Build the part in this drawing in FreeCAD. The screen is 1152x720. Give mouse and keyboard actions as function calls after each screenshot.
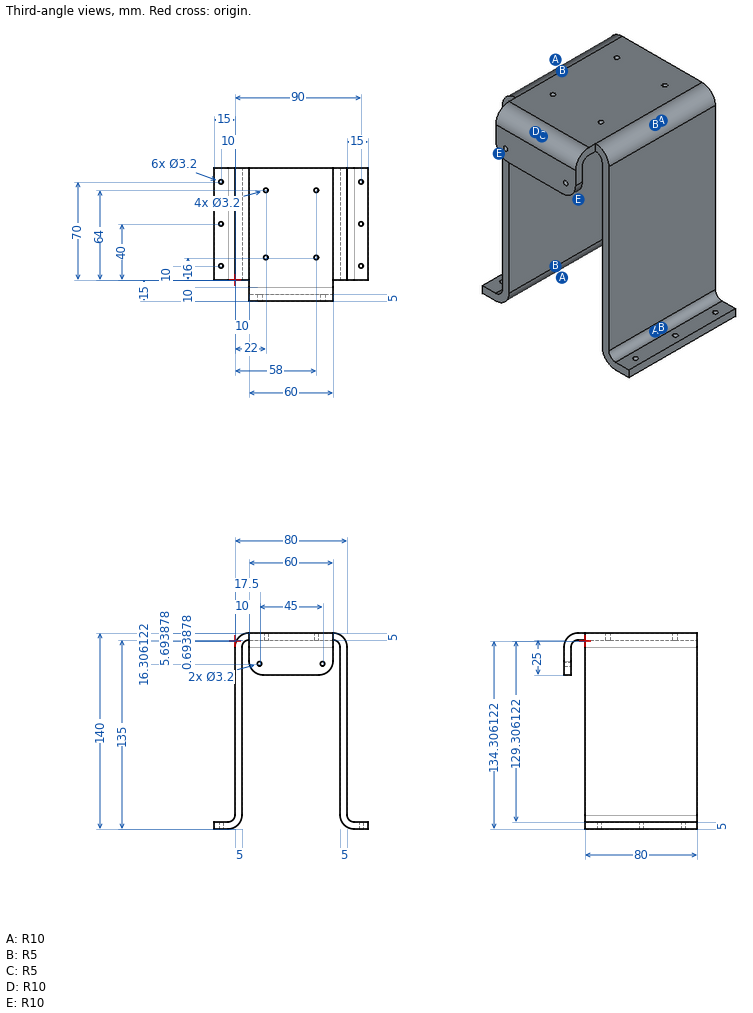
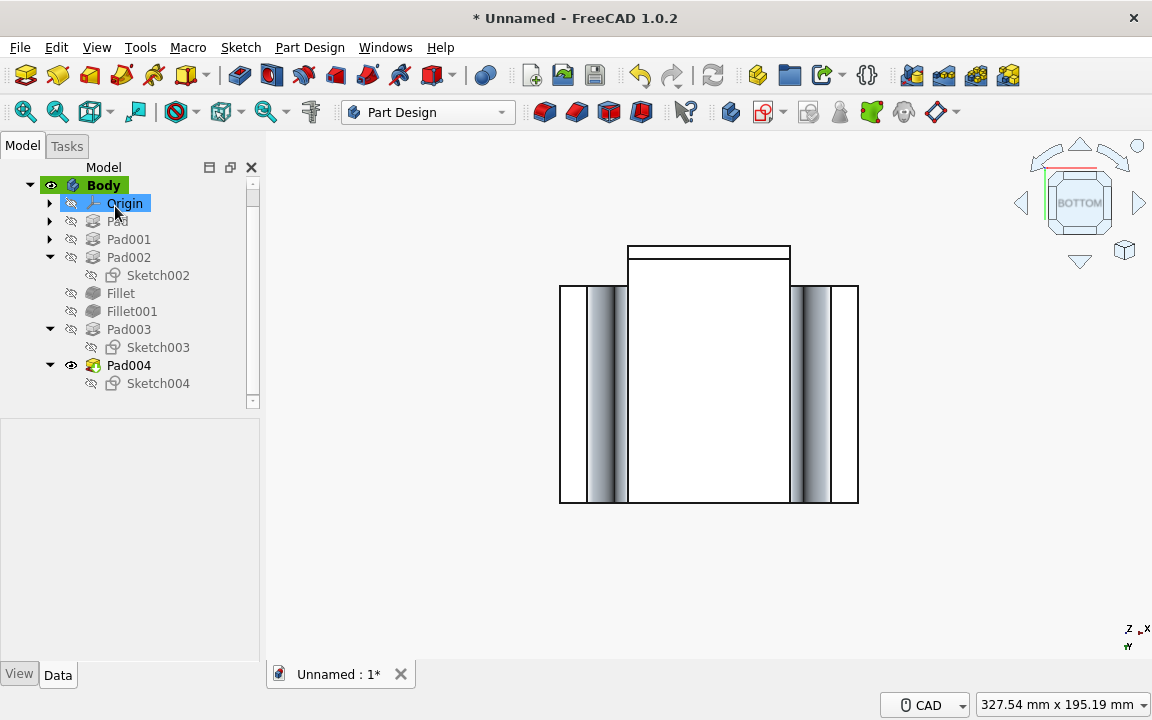
key(0)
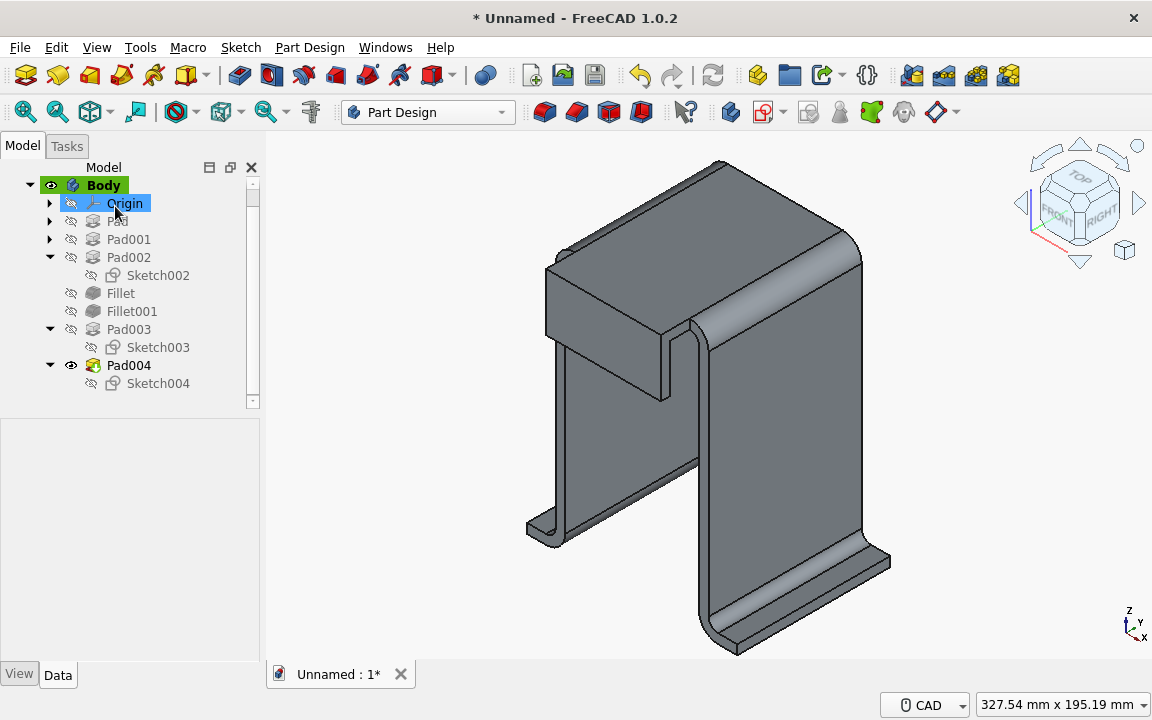
click(26, 112)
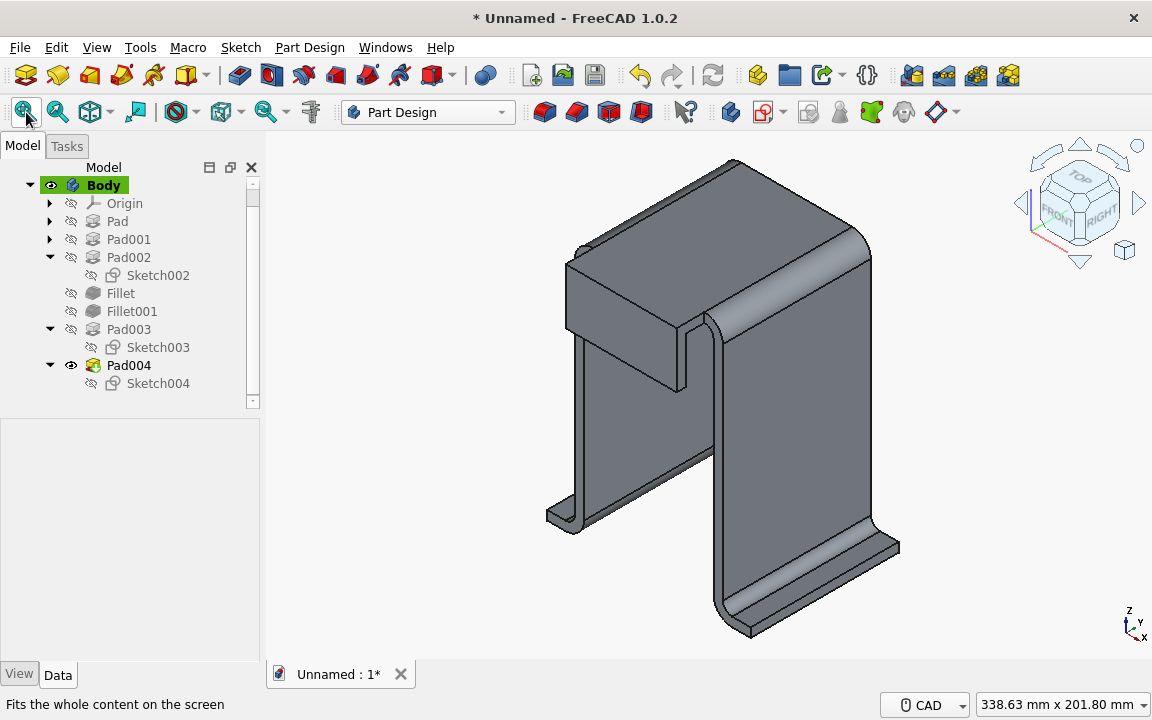
key(2)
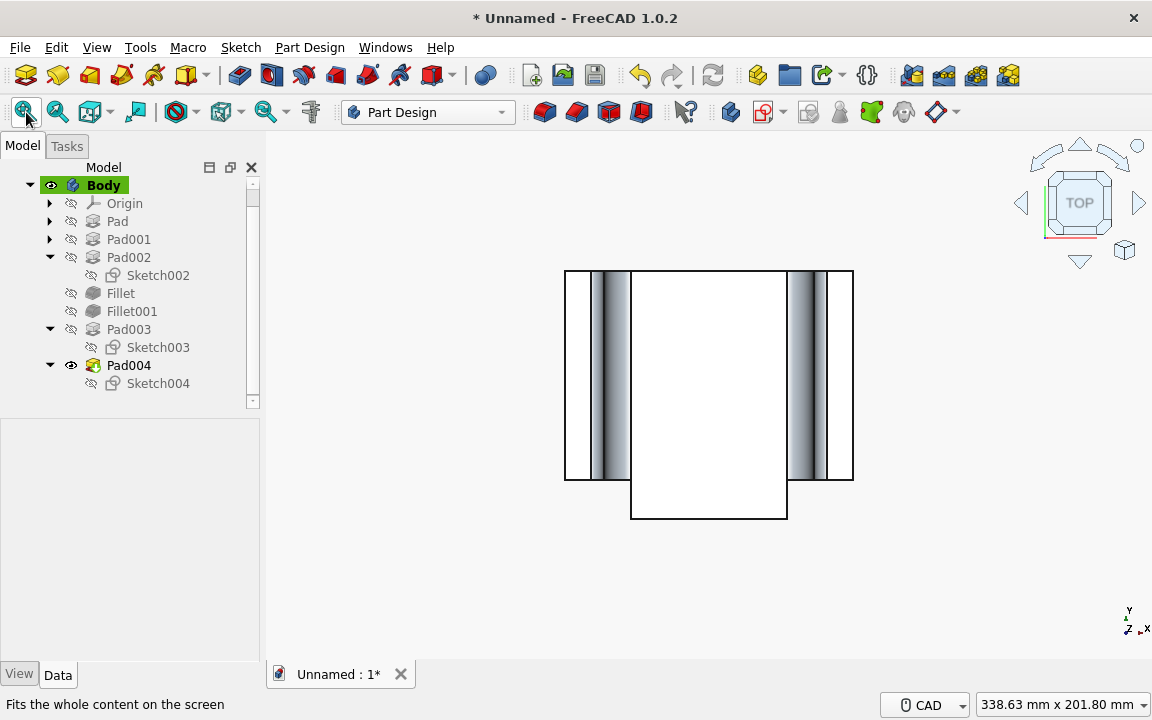
key(1)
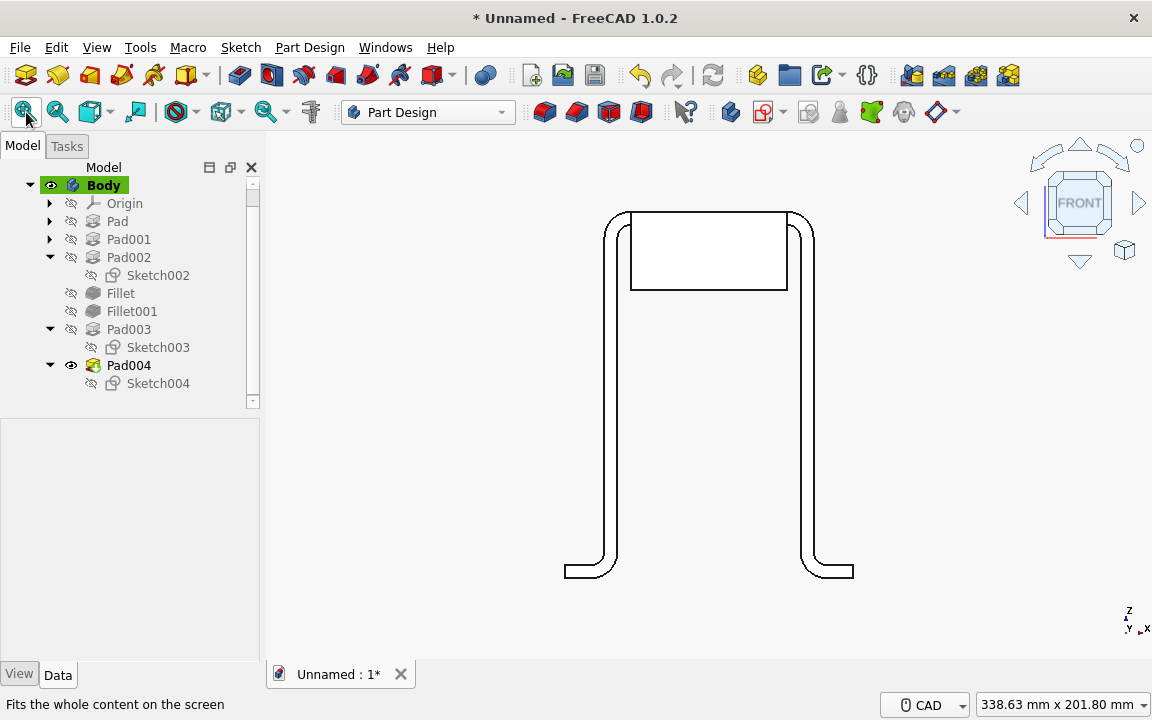
key(3)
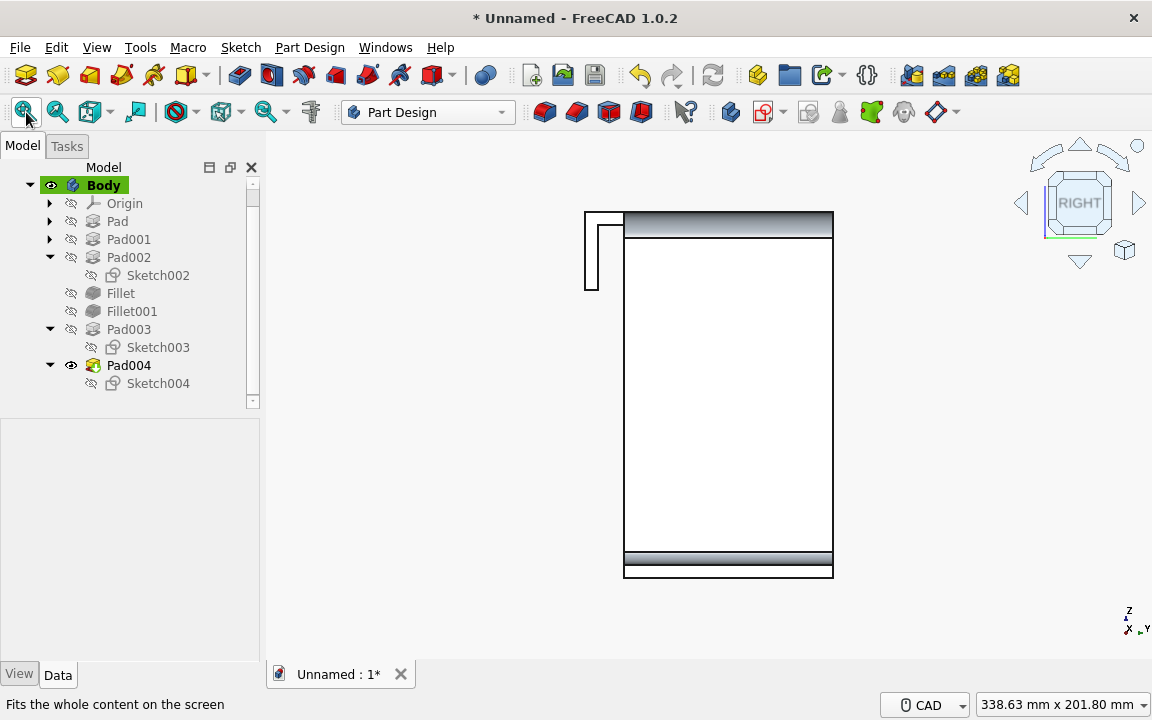
key(5)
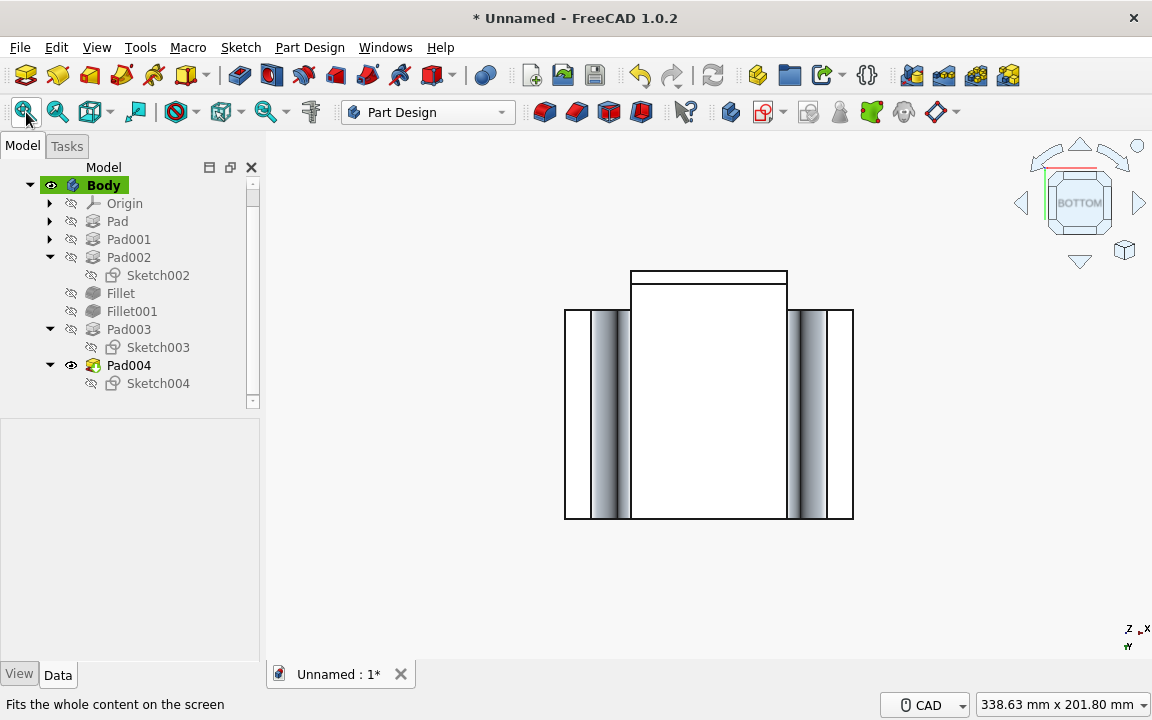
key(4)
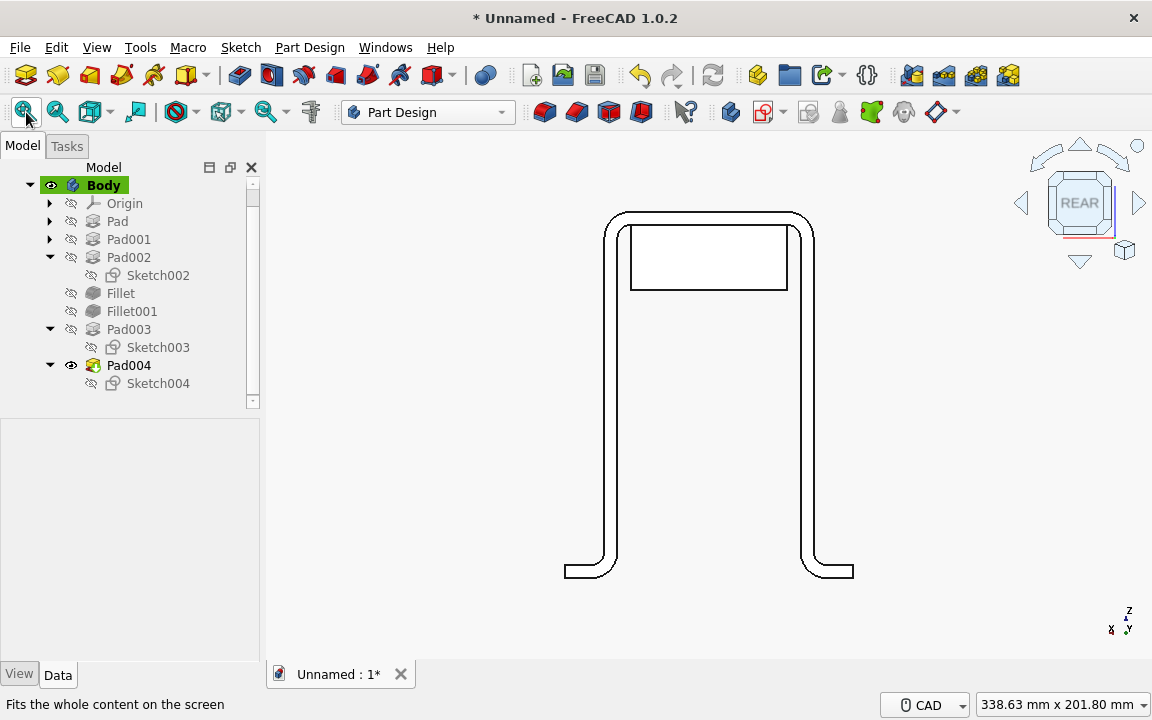
key(6)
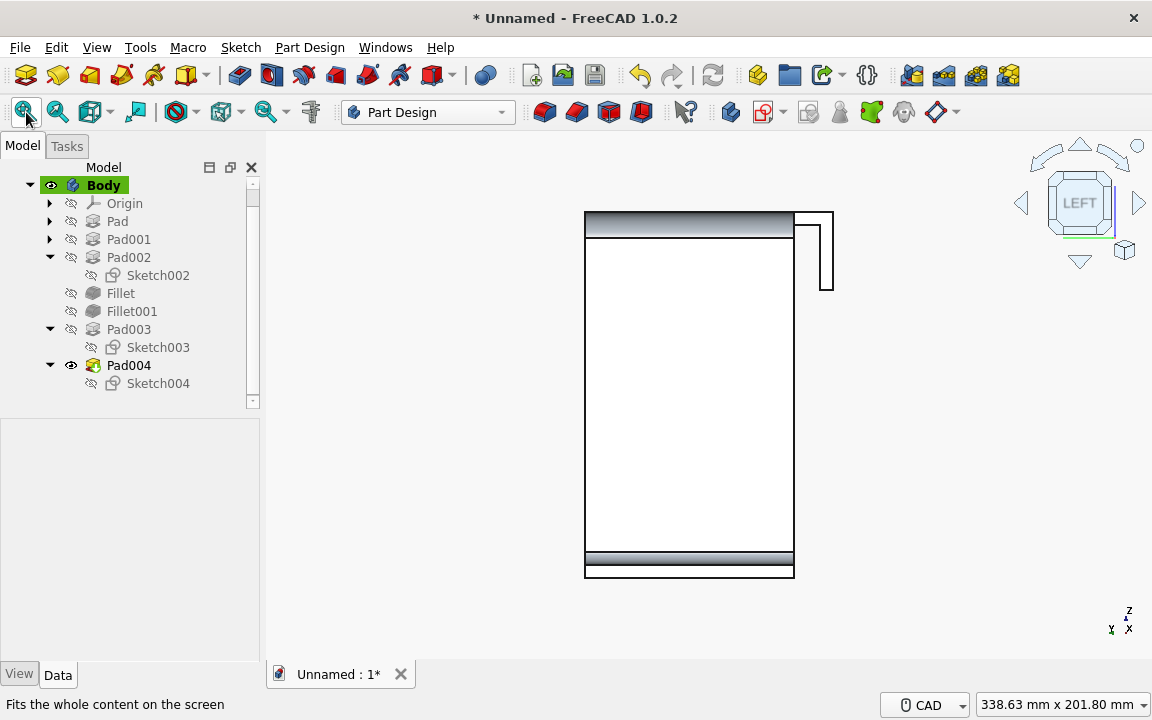
key(v)
key(3)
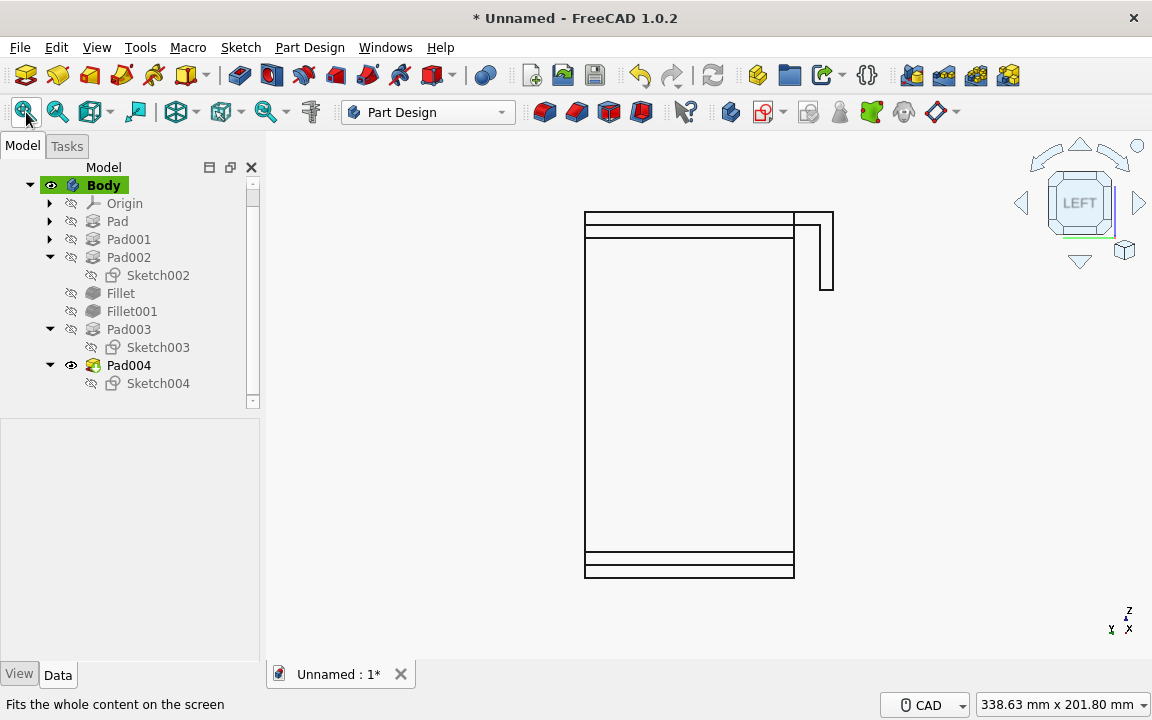
key(0)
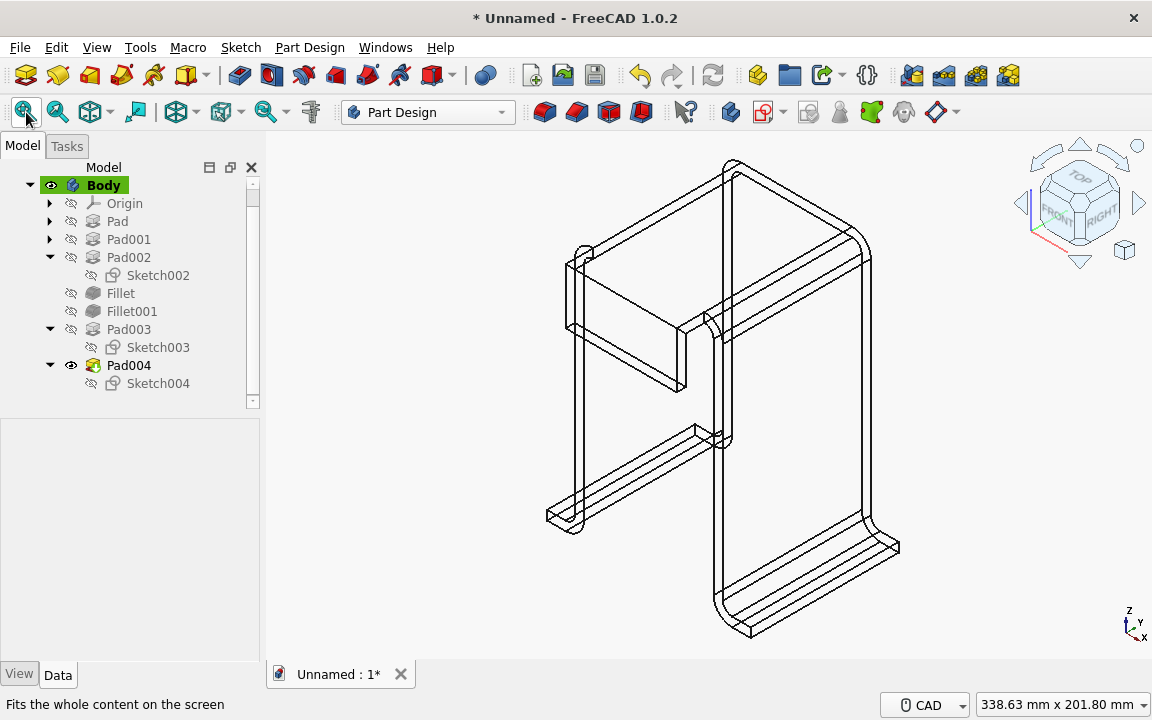
key(2)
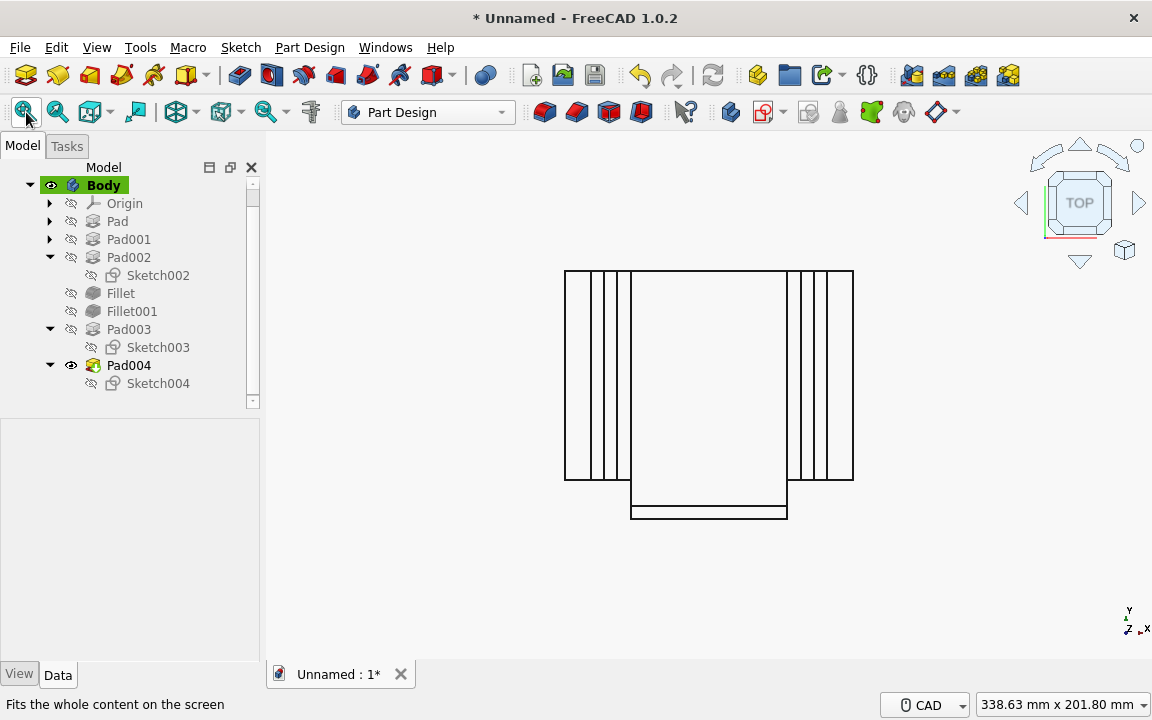
click(709, 505)